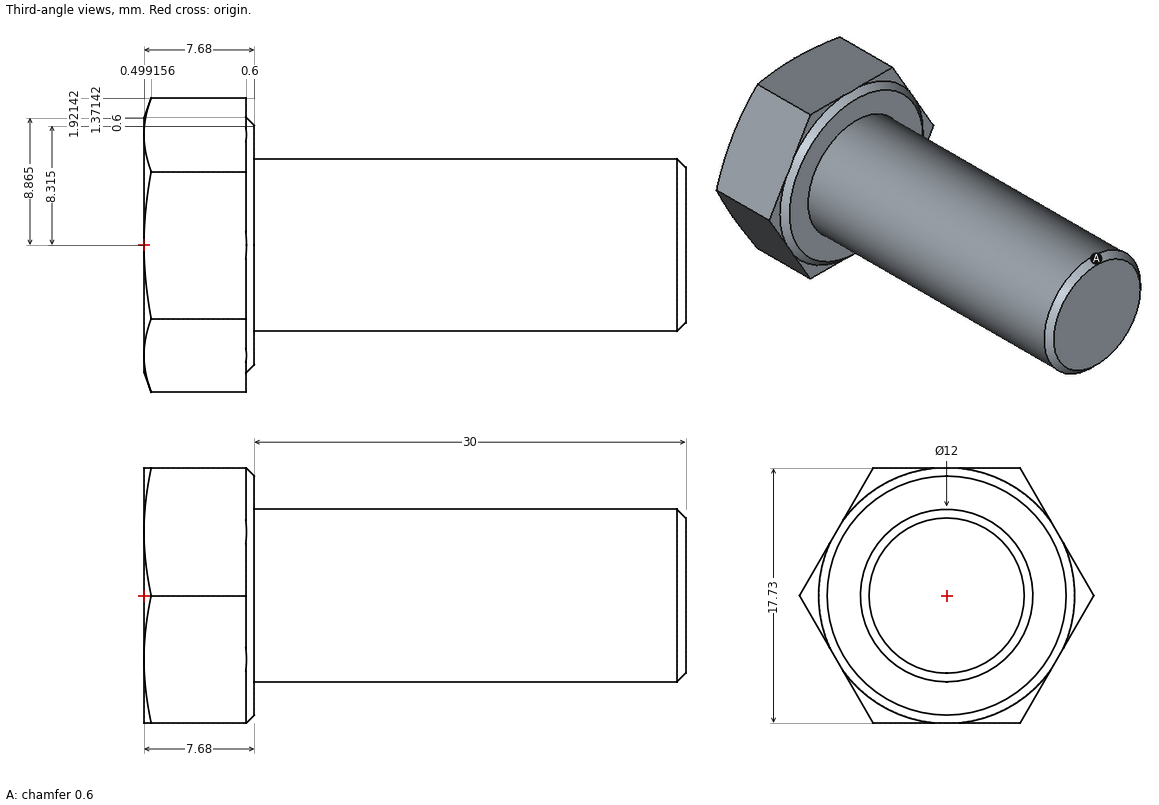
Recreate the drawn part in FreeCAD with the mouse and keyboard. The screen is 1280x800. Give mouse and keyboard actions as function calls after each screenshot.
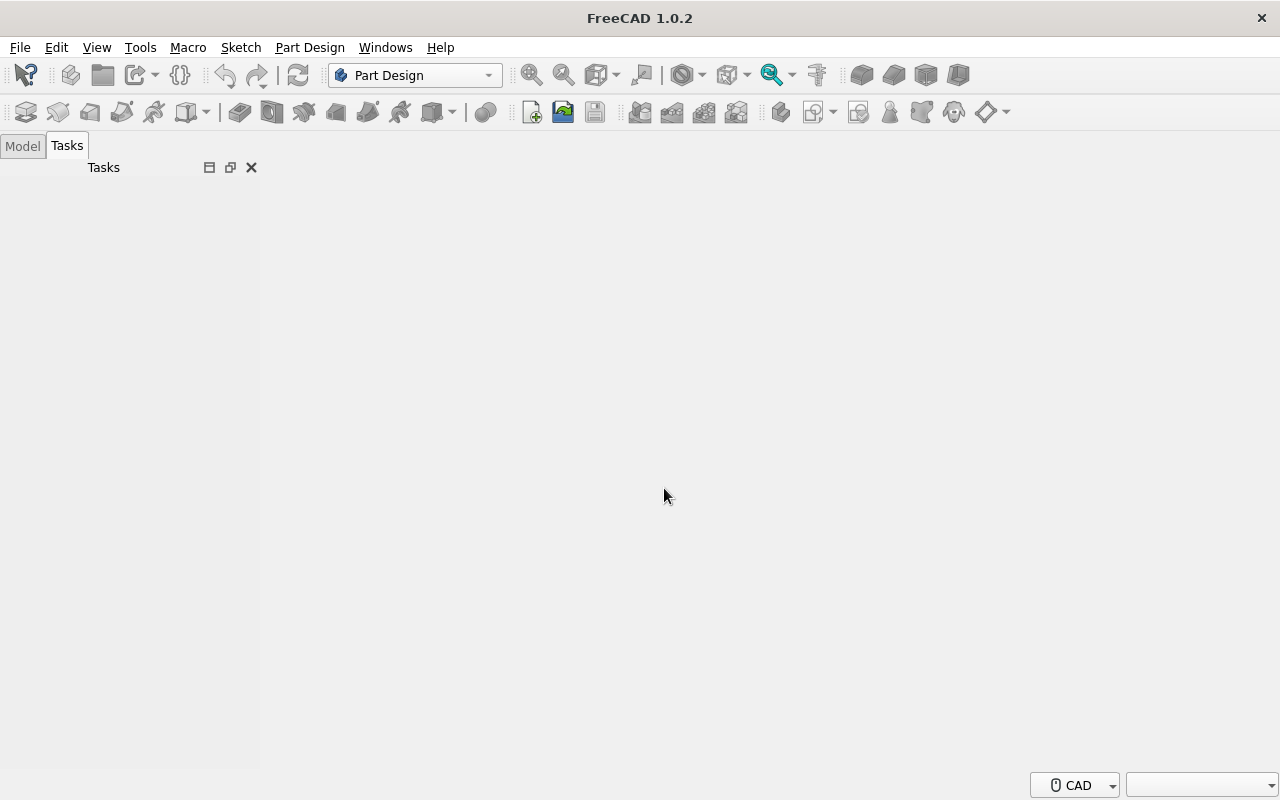
click(532, 112)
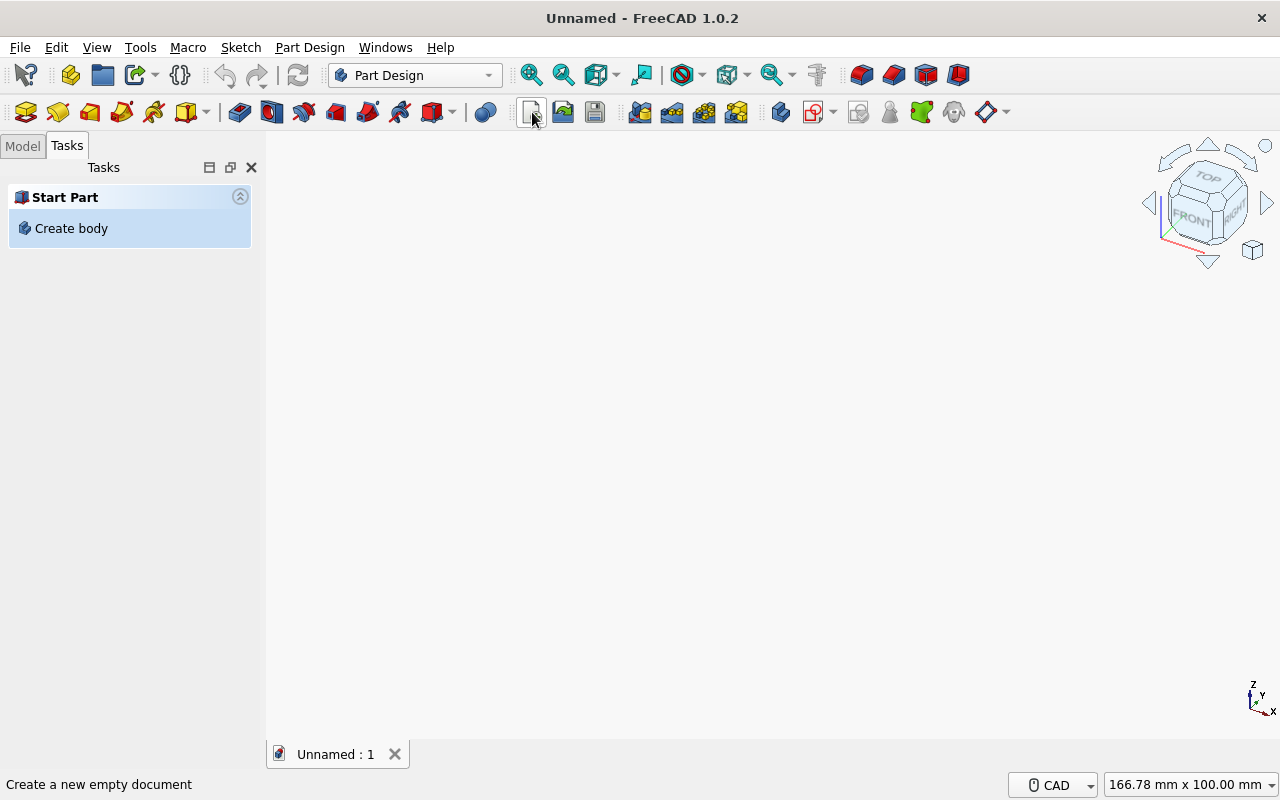
click(814, 112)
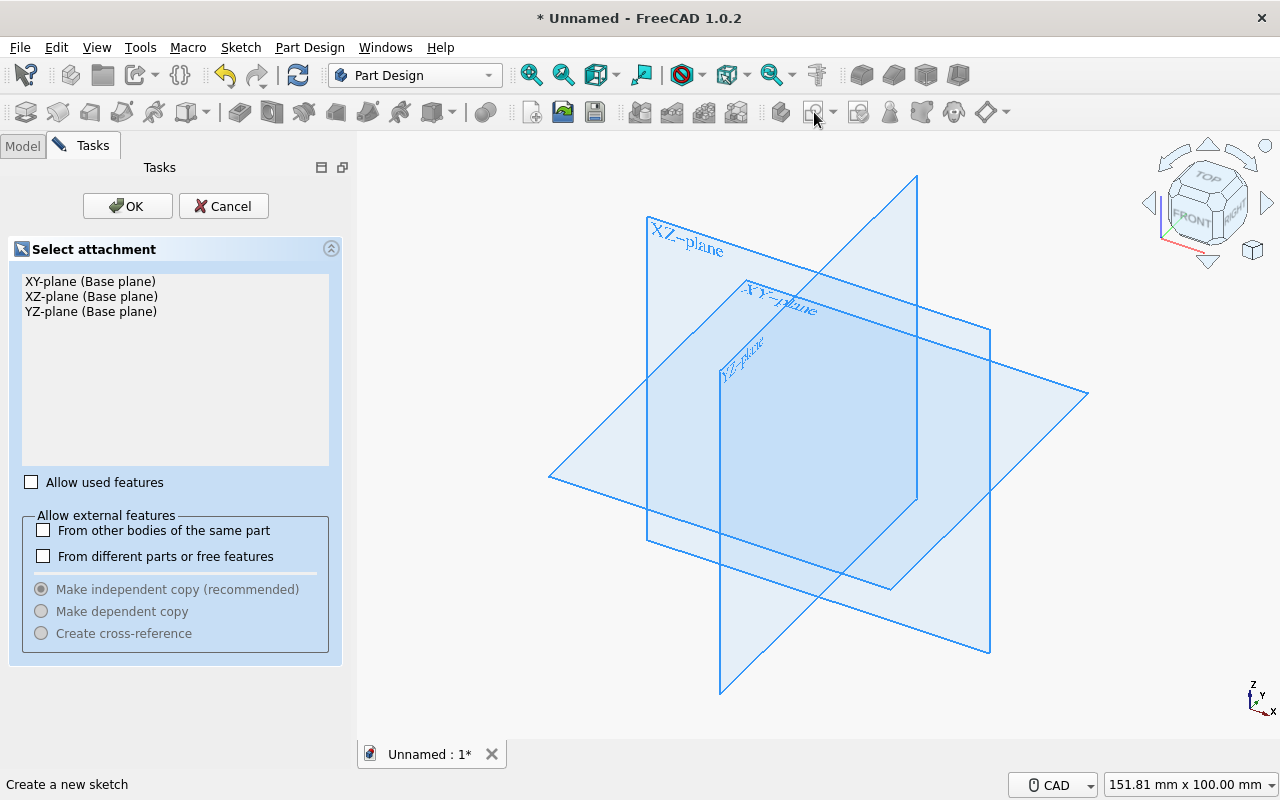
click(82, 312)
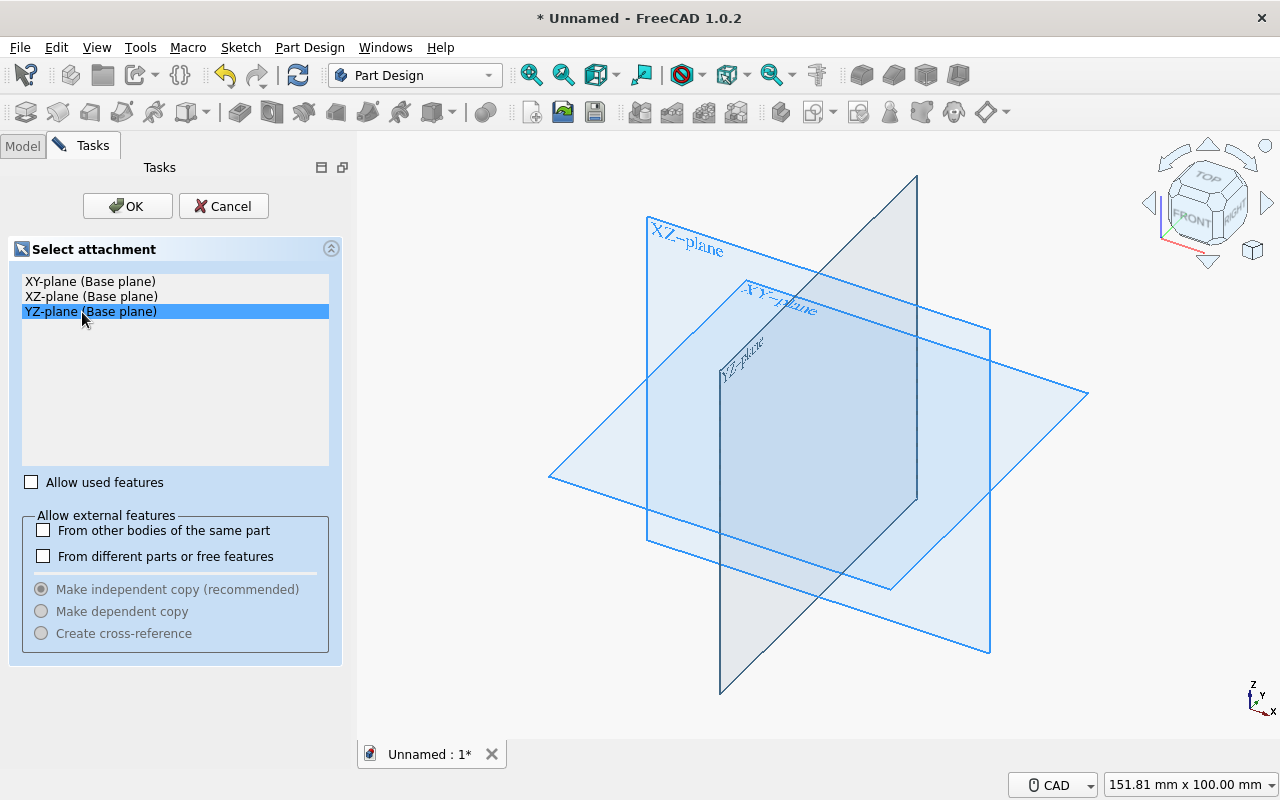
click(128, 206)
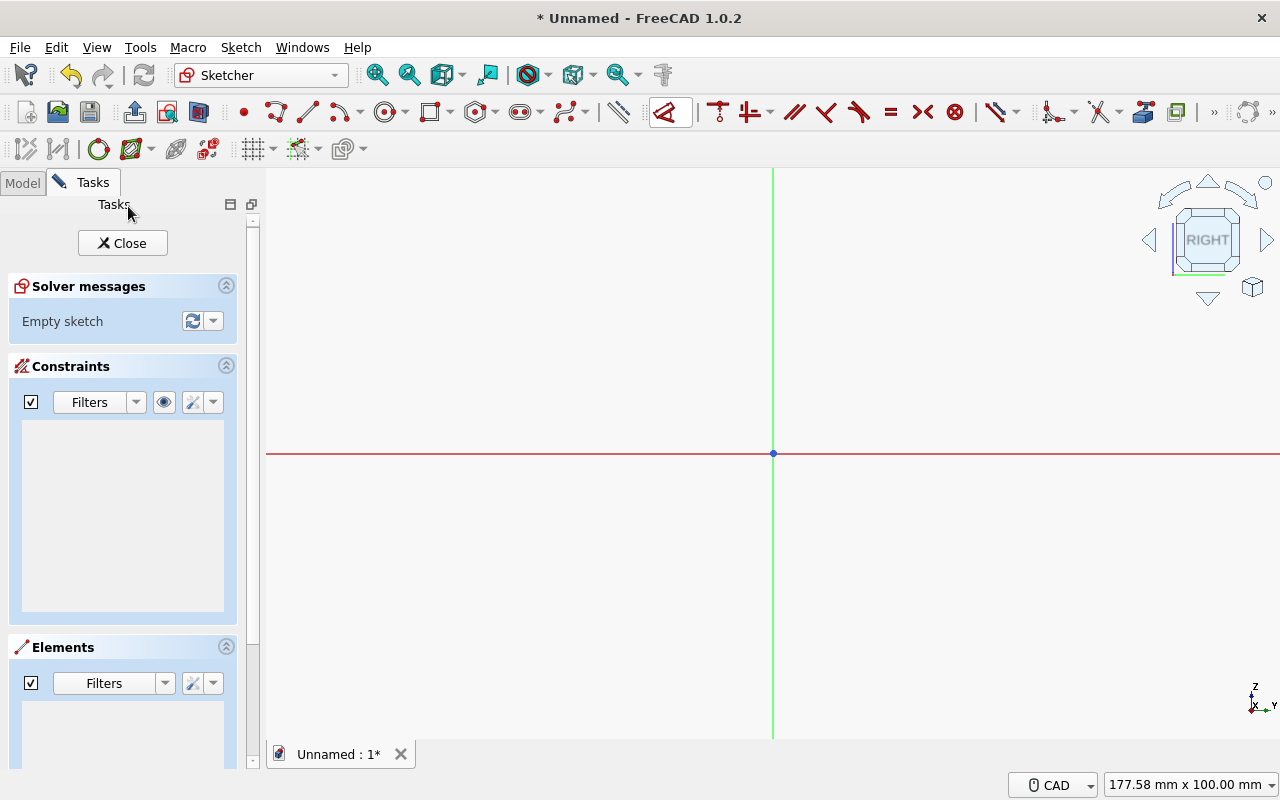
scroll(803, 454, up, 6)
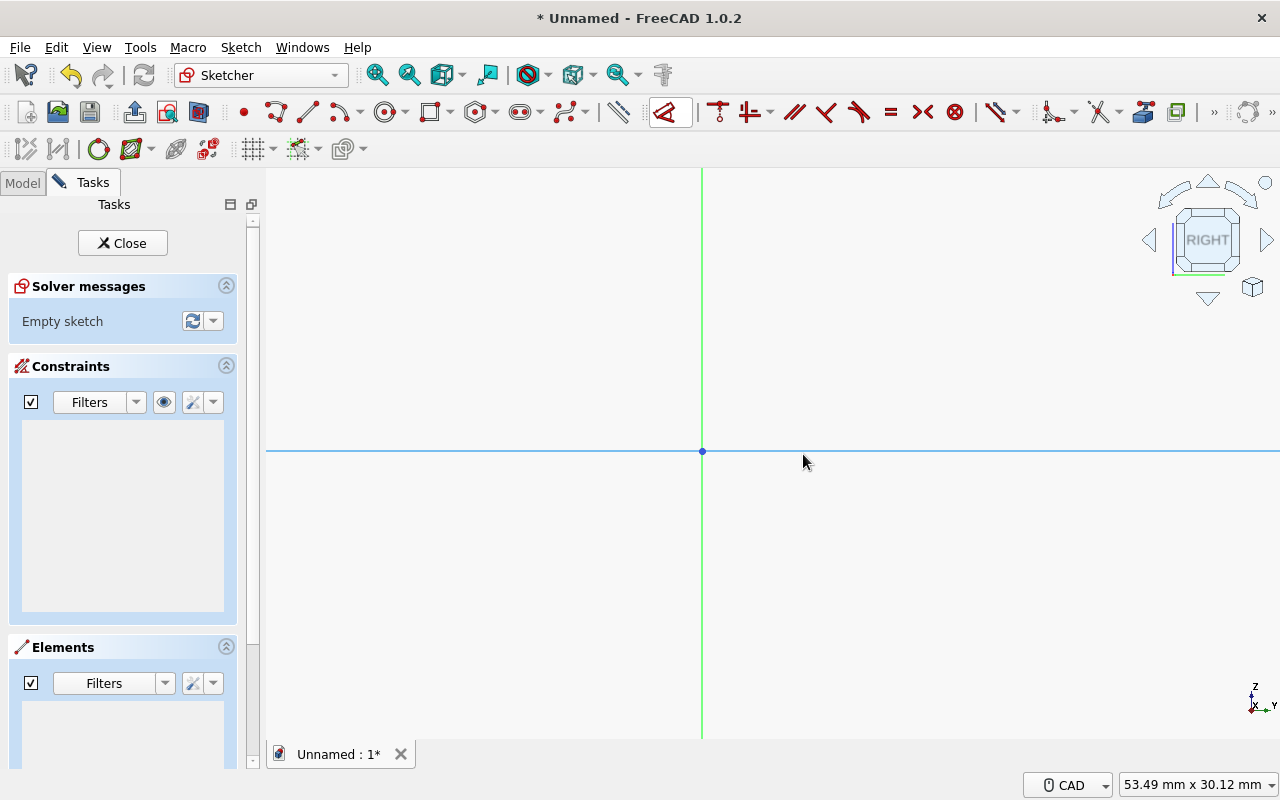
click(476, 112)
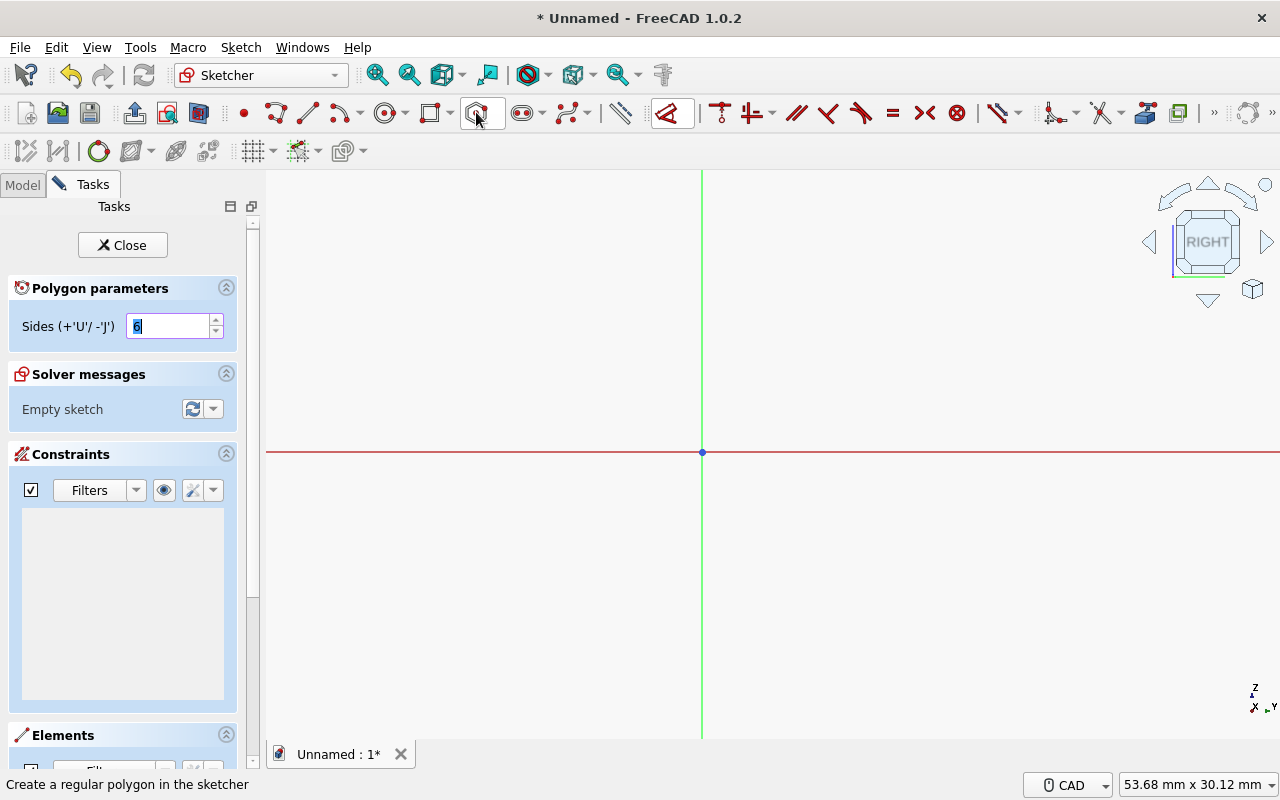
click(702, 452)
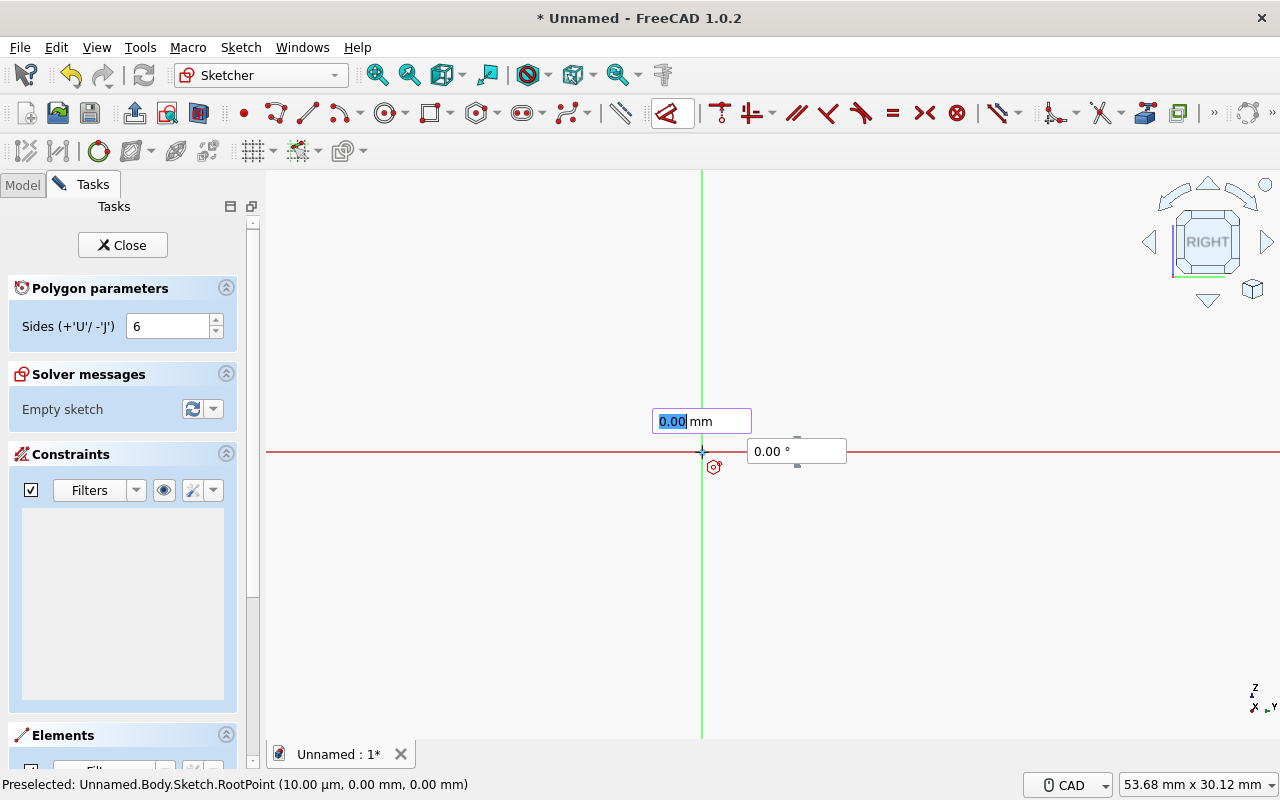
click(896, 452)
key(Escape)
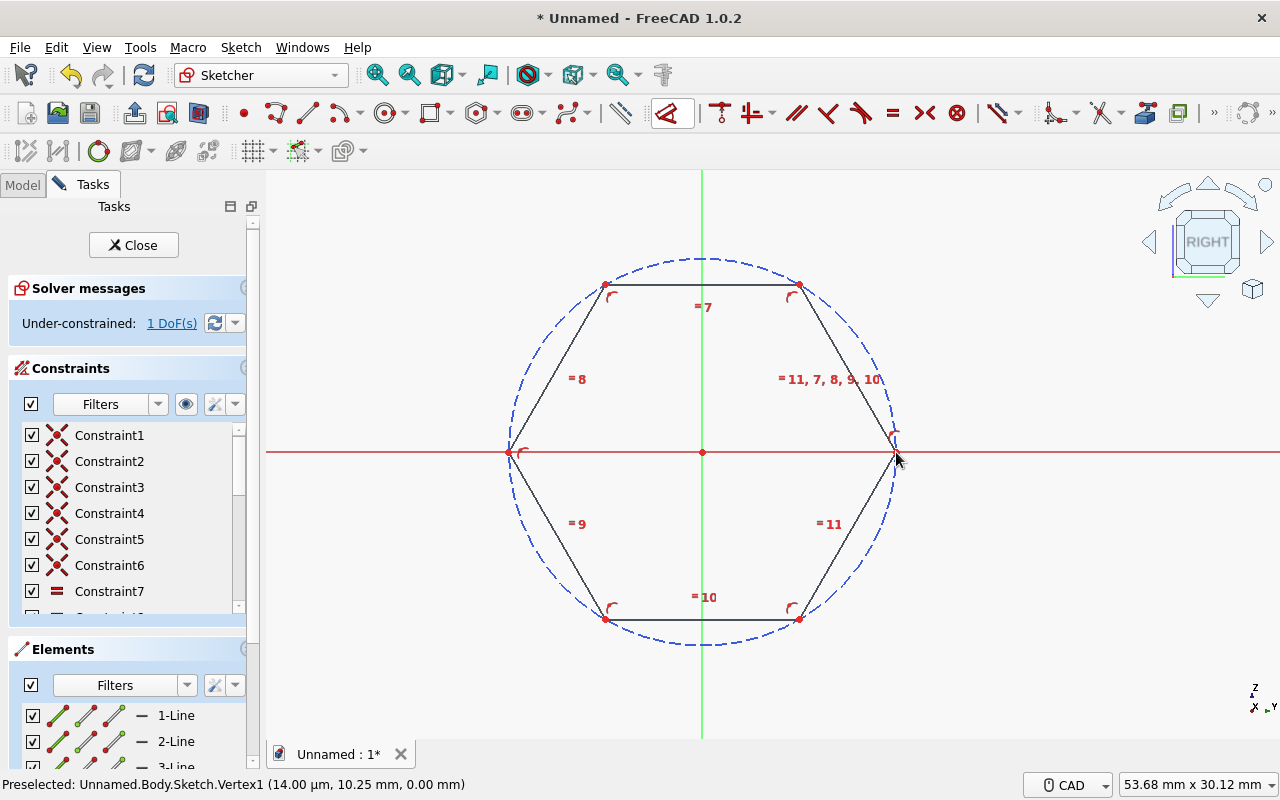
click(666, 114)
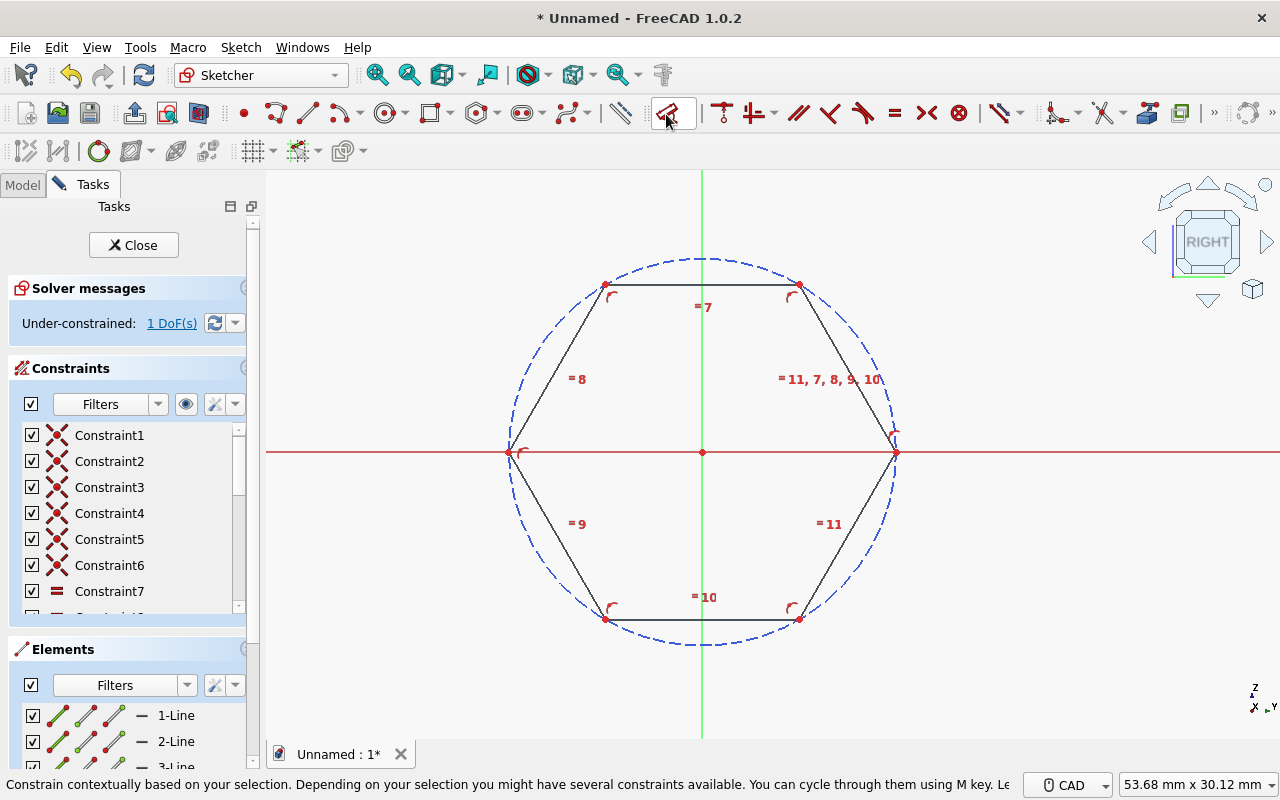
click(606, 620)